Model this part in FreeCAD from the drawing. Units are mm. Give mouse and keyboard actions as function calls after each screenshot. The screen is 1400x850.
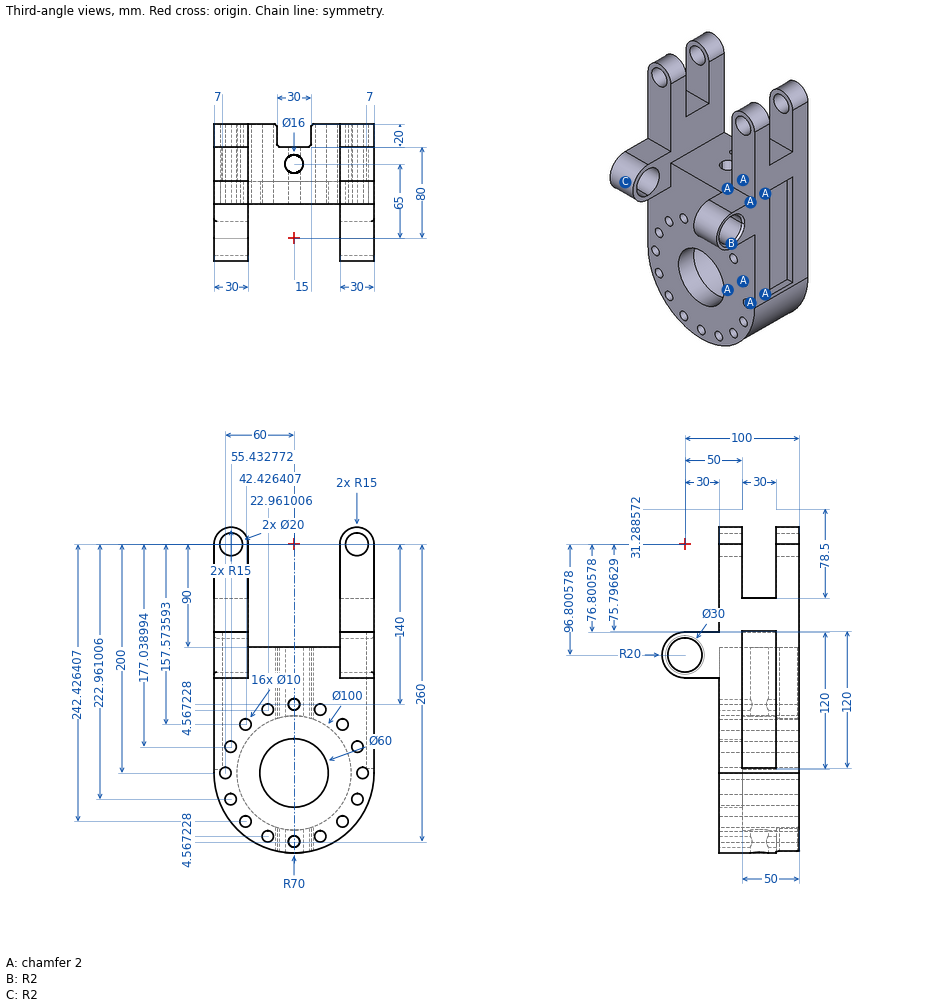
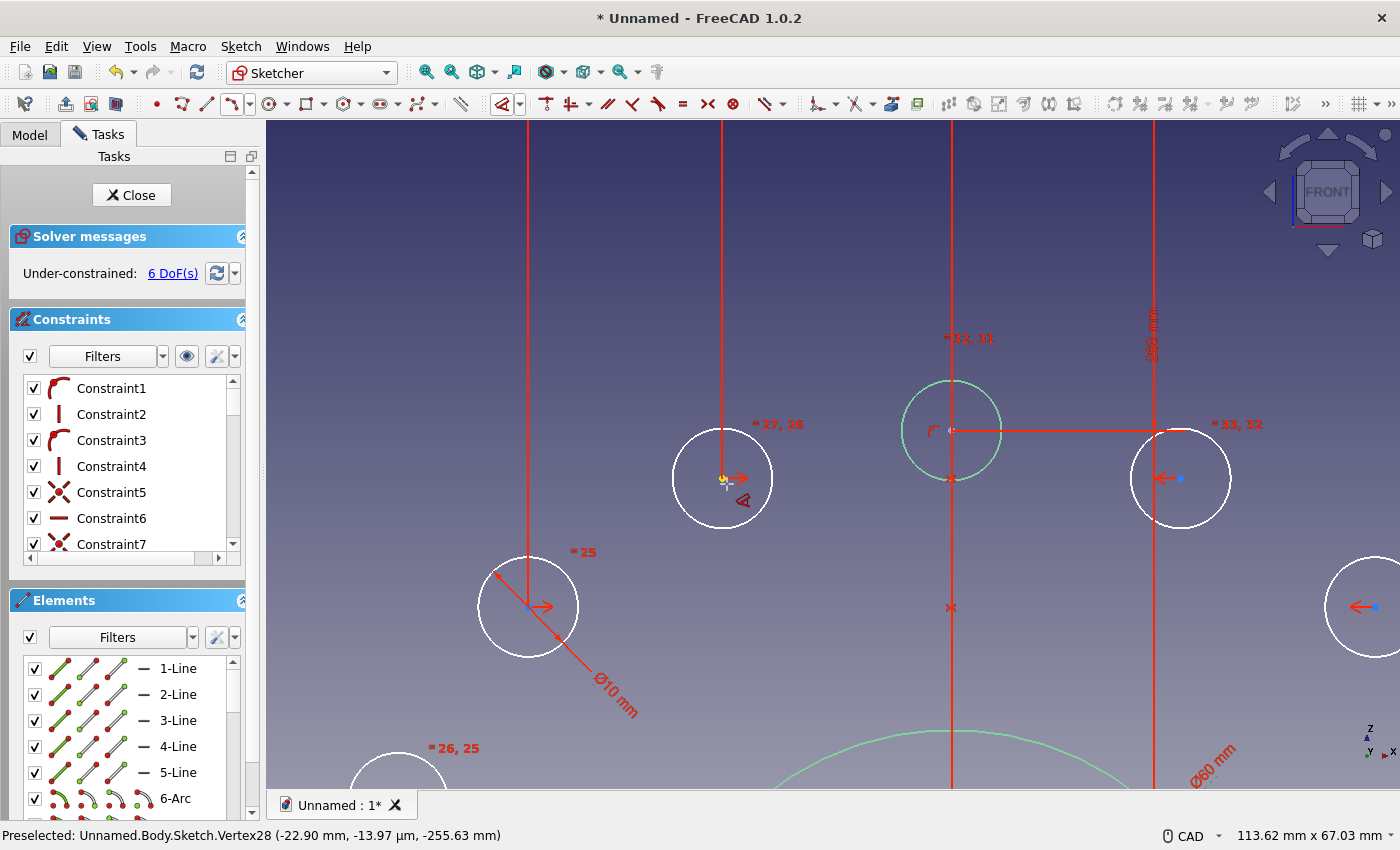
click(722, 478)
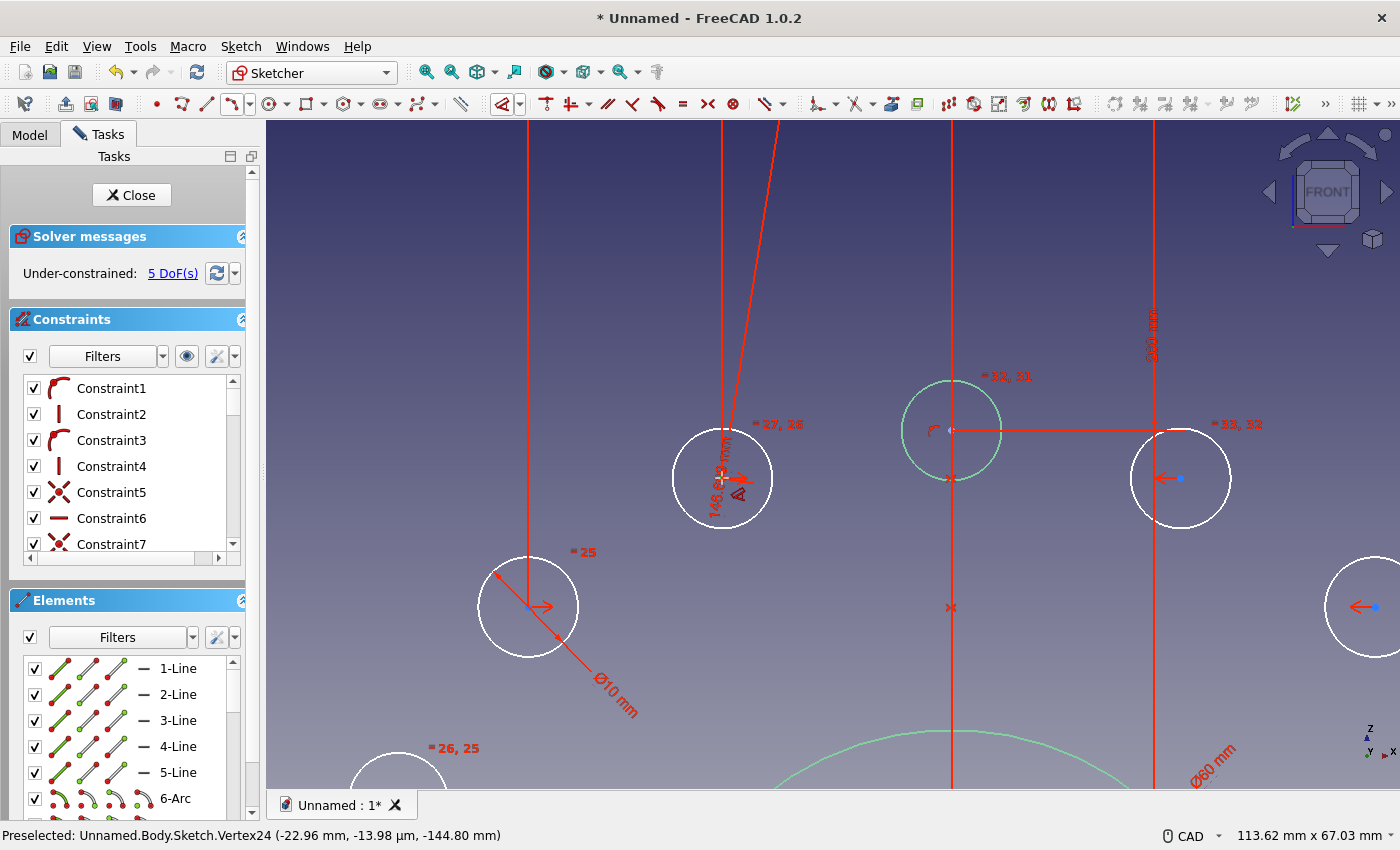
click(952, 431)
click(688, 465)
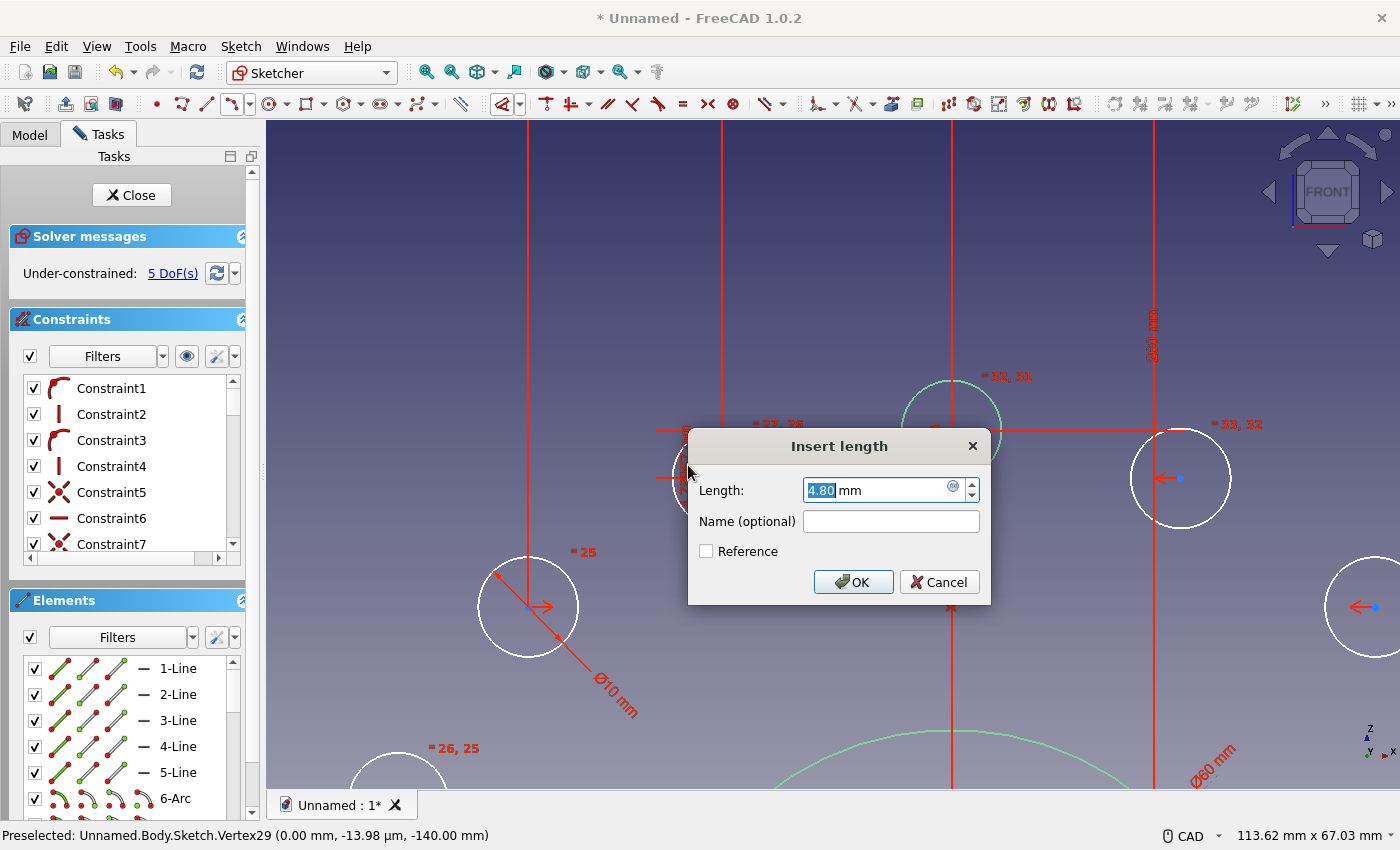
text(4.567228)
key(Return)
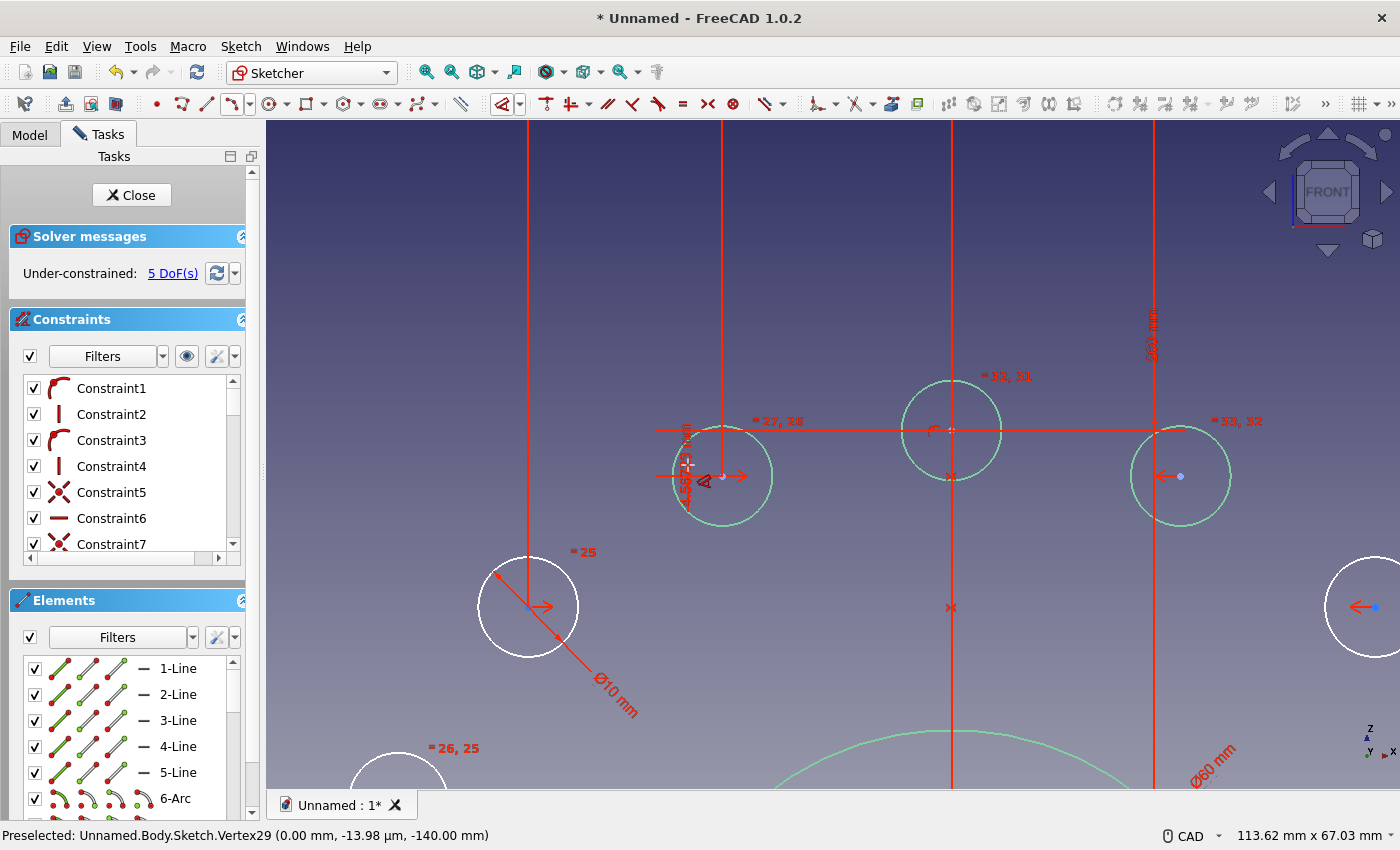
scroll(727, 484, down, 9)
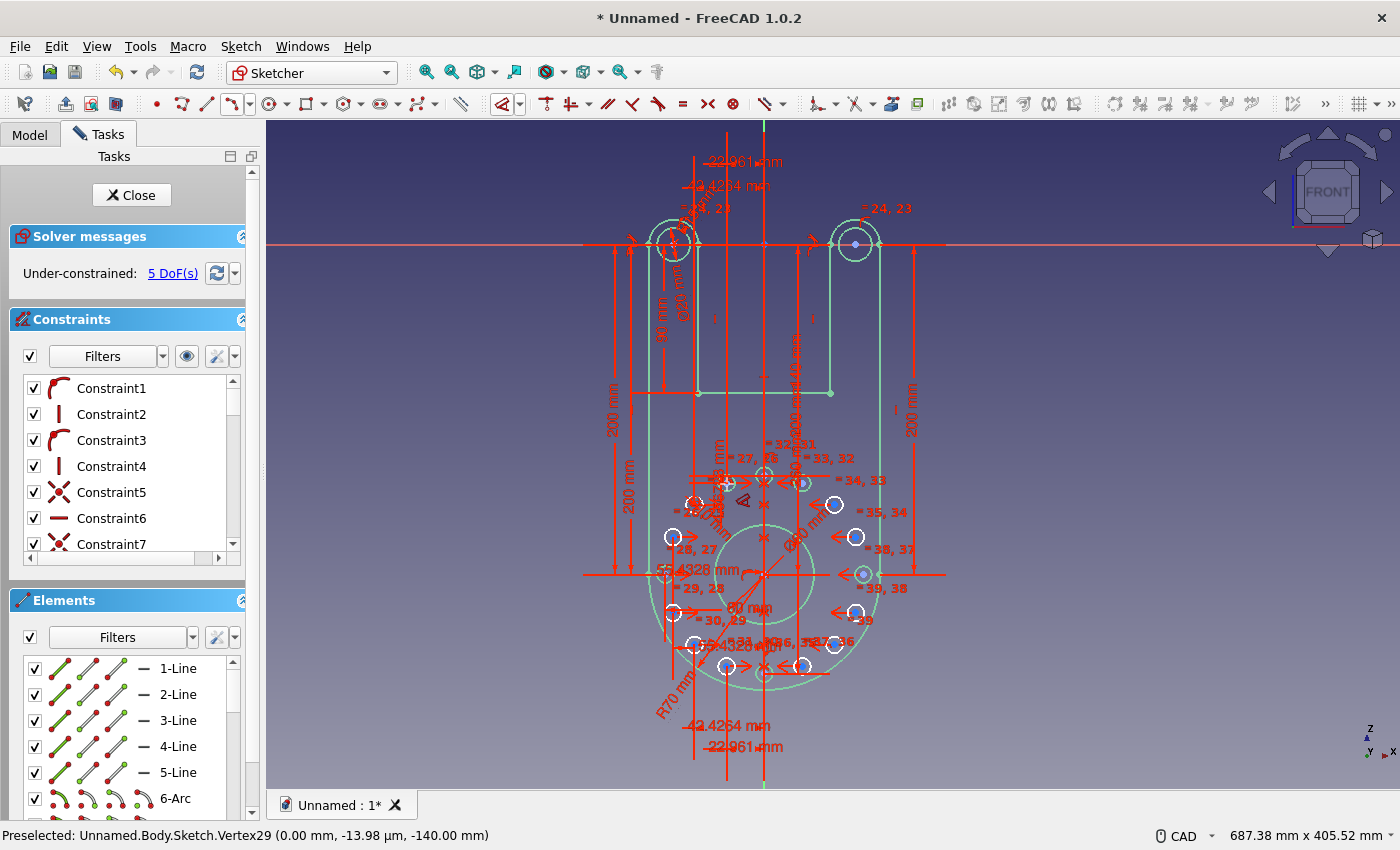
scroll(727, 666, up, 9)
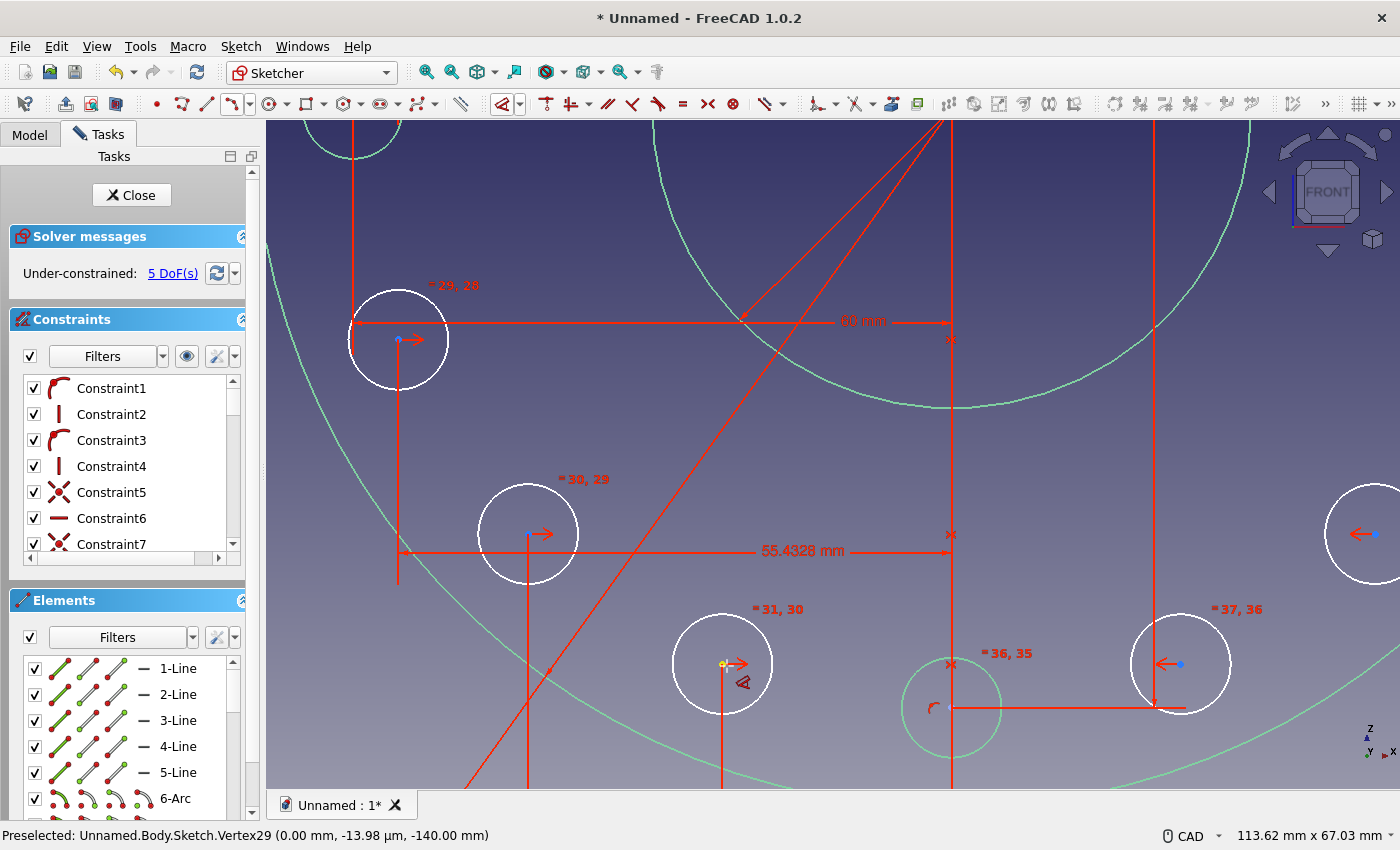
click(722, 664)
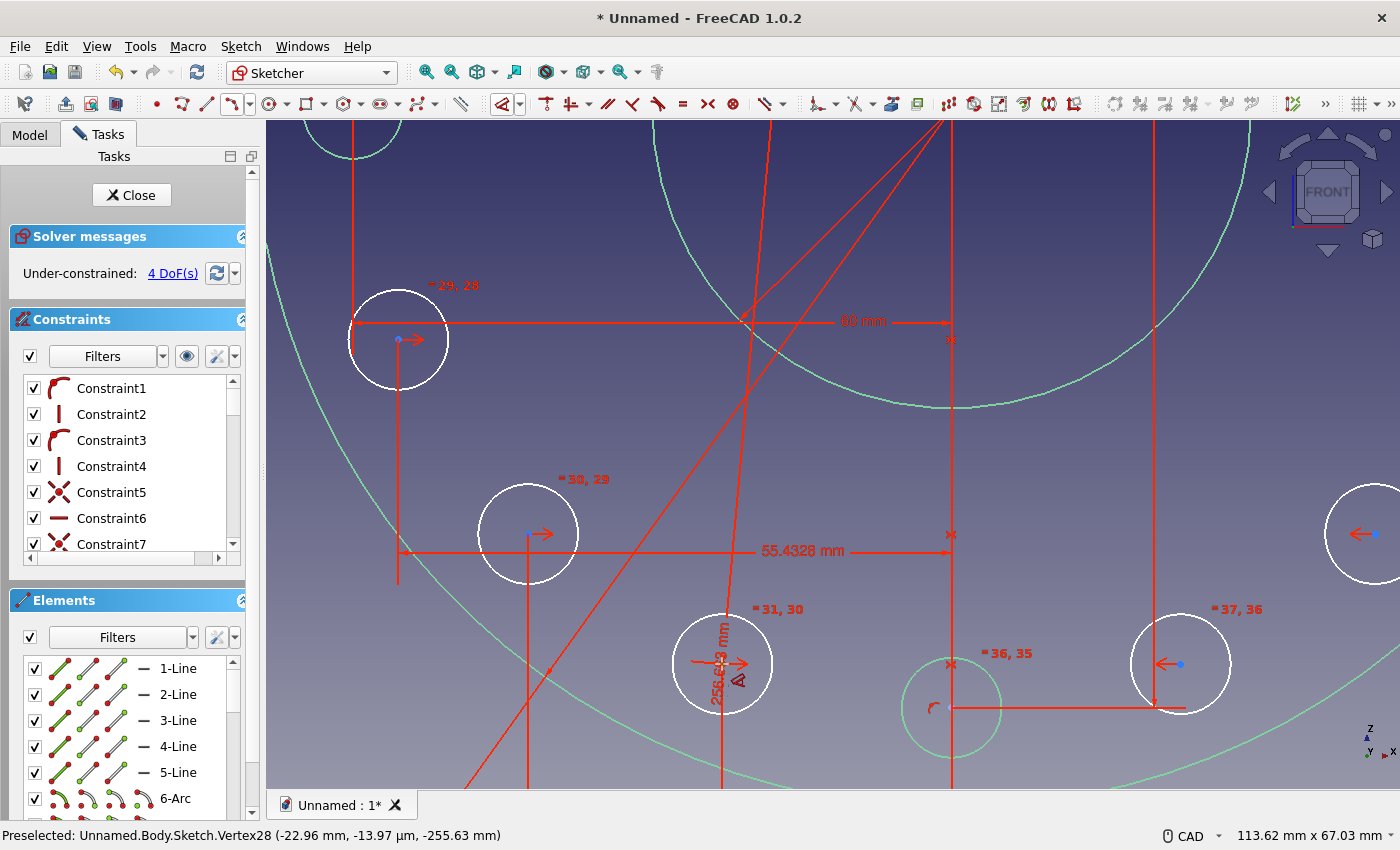
click(952, 708)
click(688, 676)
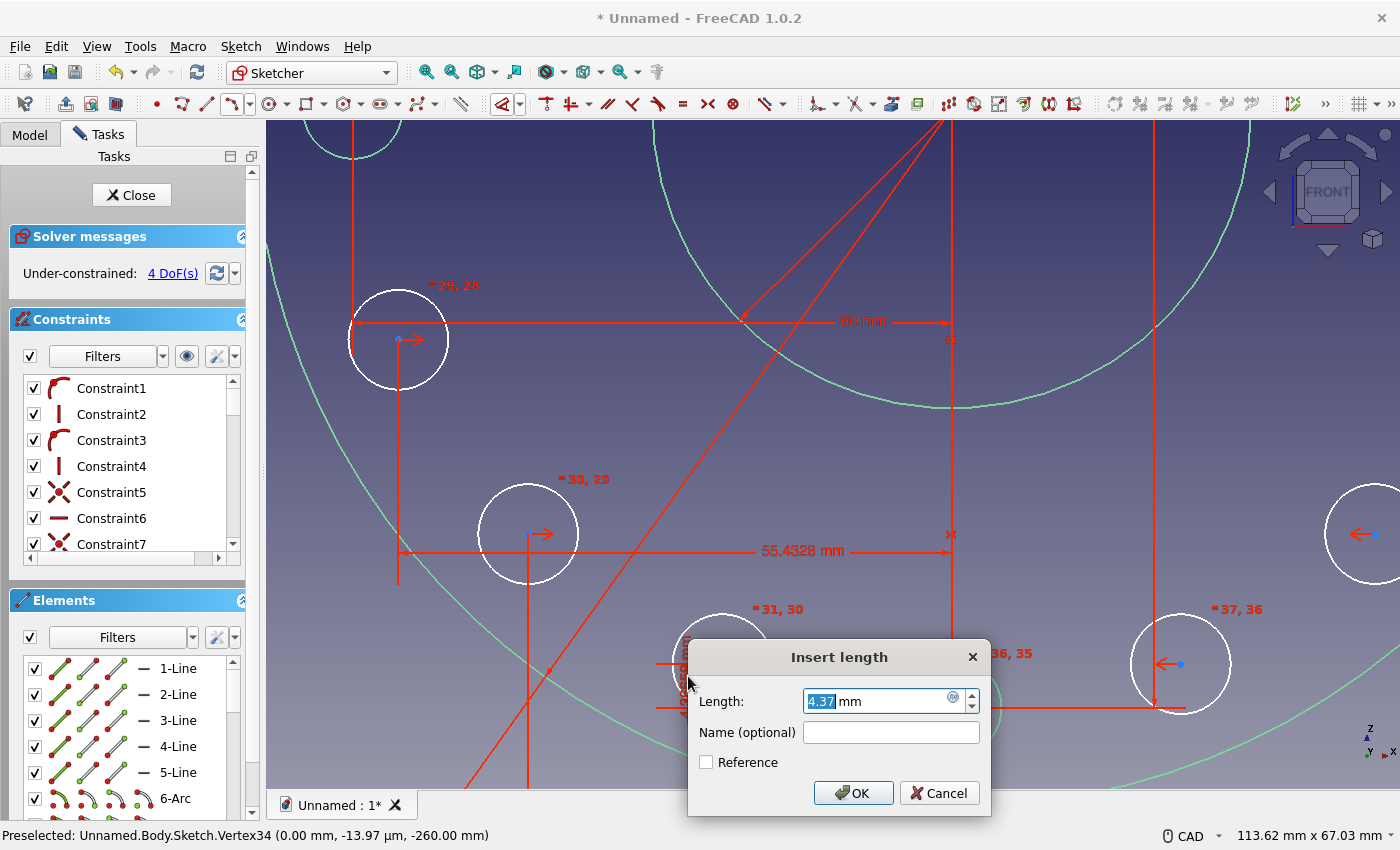
text(4.567228)
key(Return)